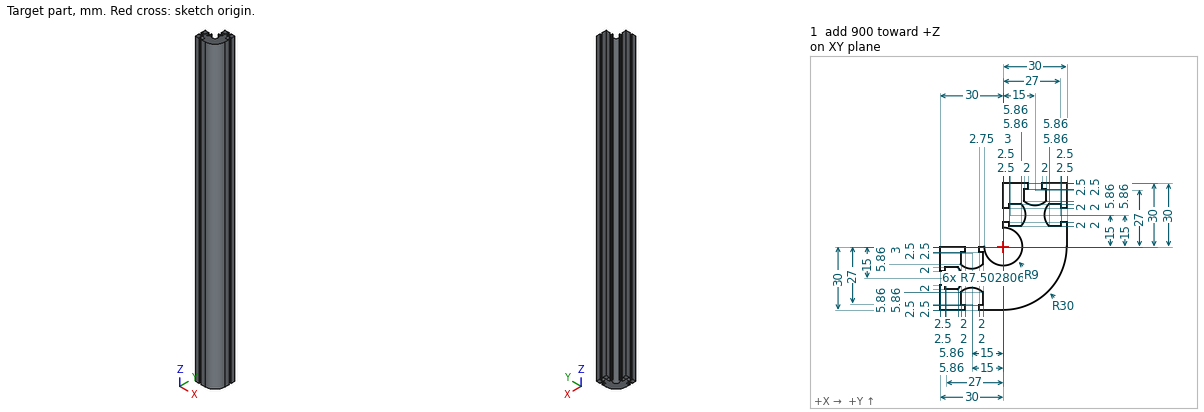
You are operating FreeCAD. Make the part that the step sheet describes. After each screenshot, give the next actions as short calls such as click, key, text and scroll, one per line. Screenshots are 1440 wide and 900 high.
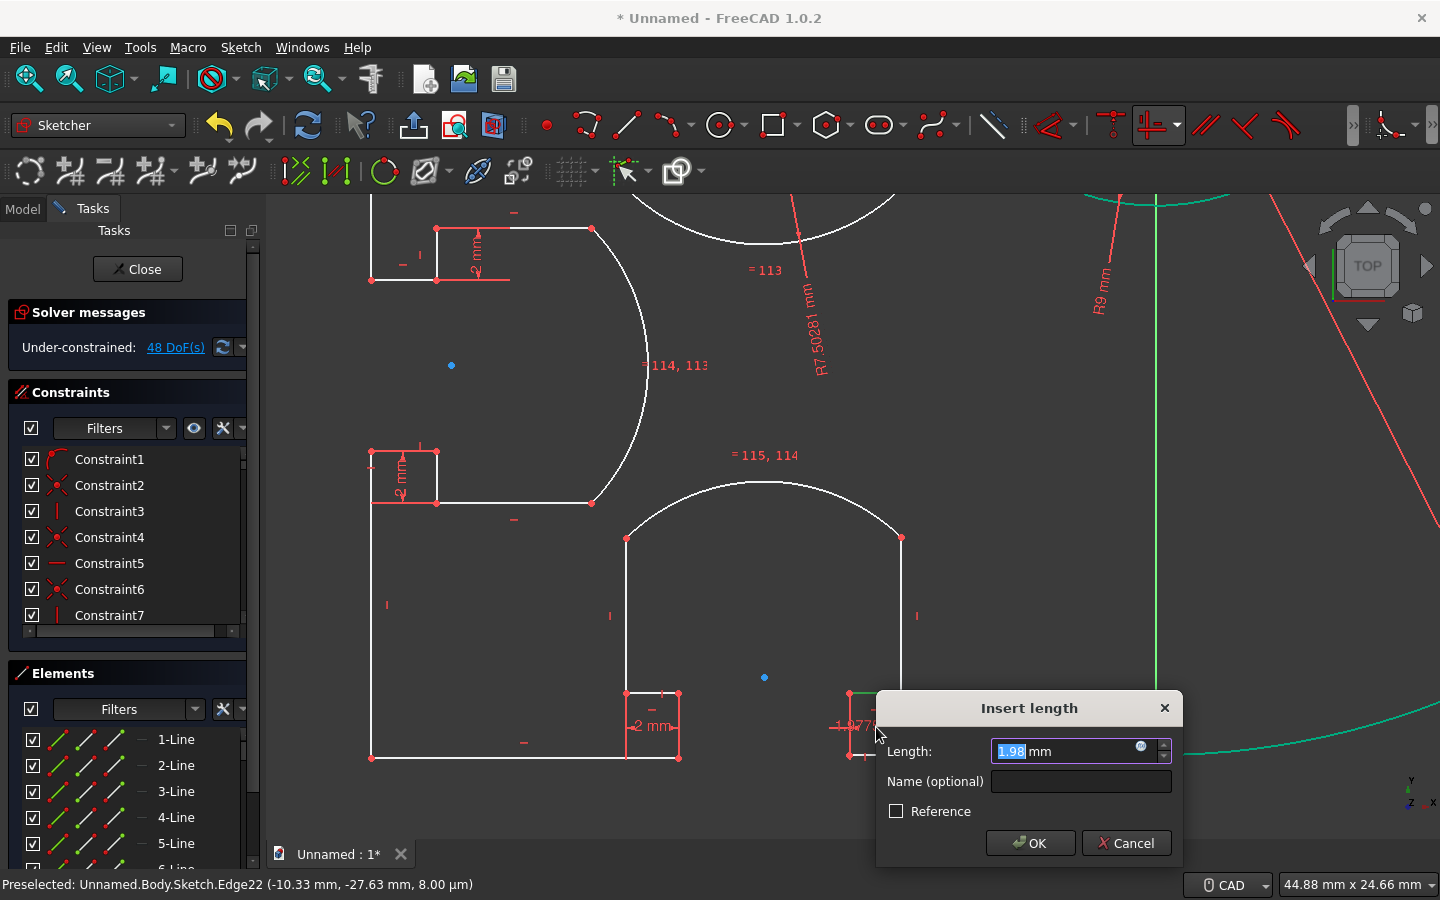
text(2)
key(Return)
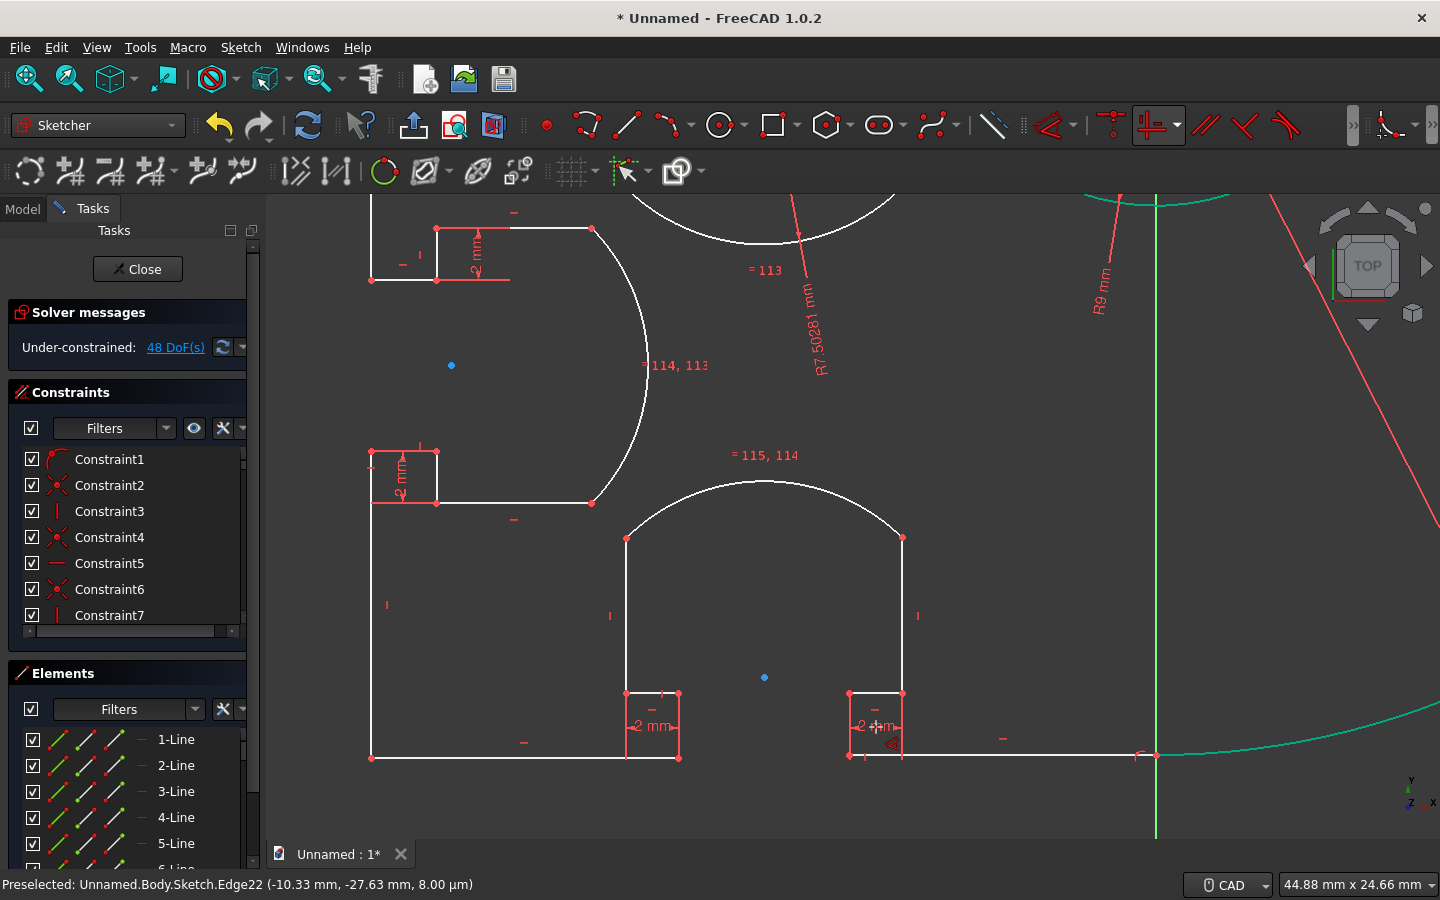
scroll(663, 695, down, 7)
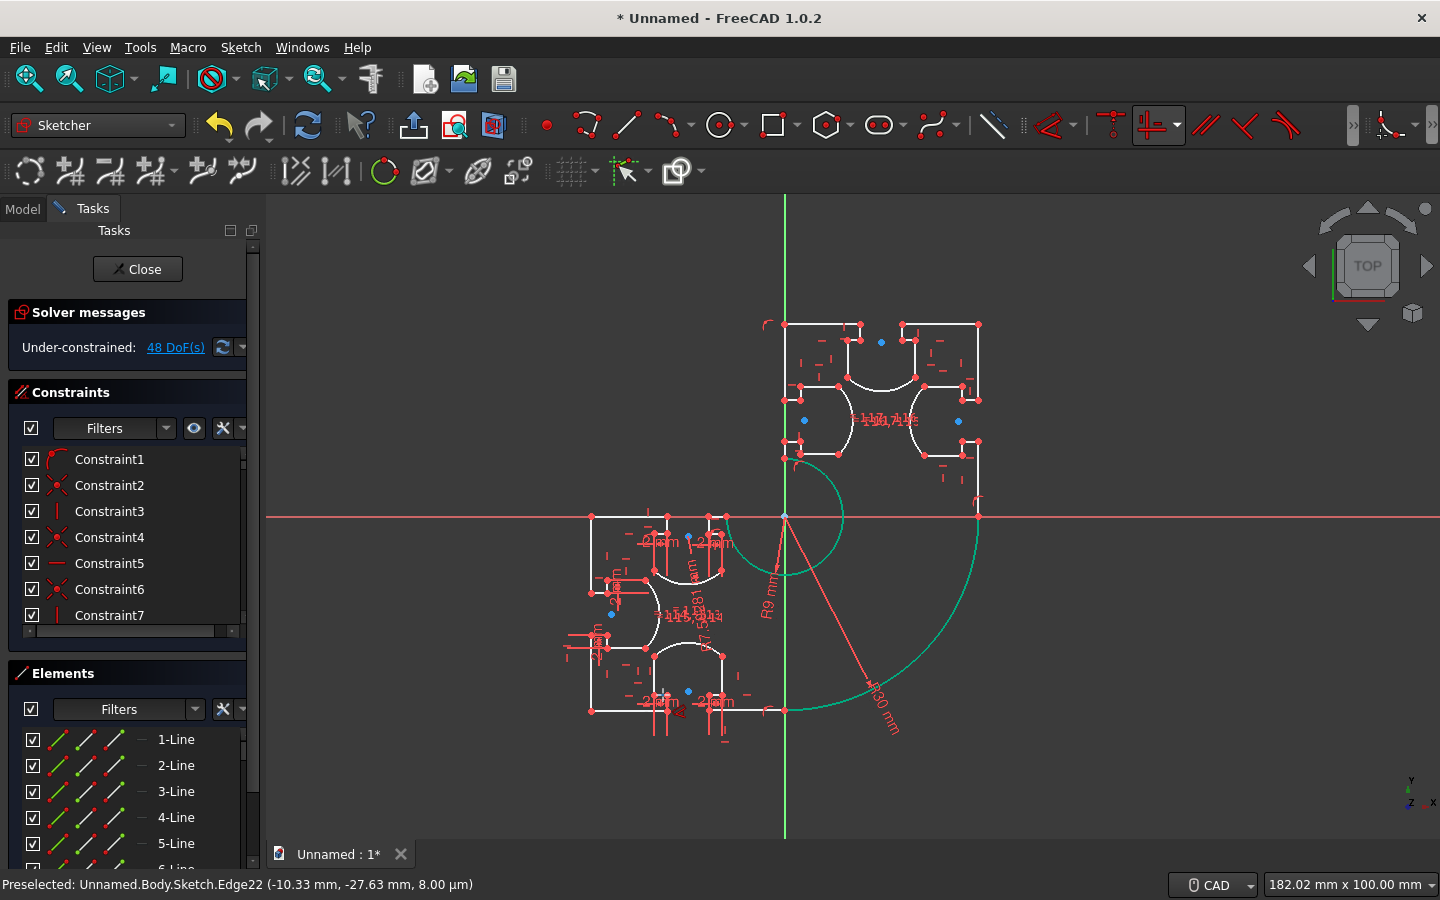
scroll(962, 446, up, 6)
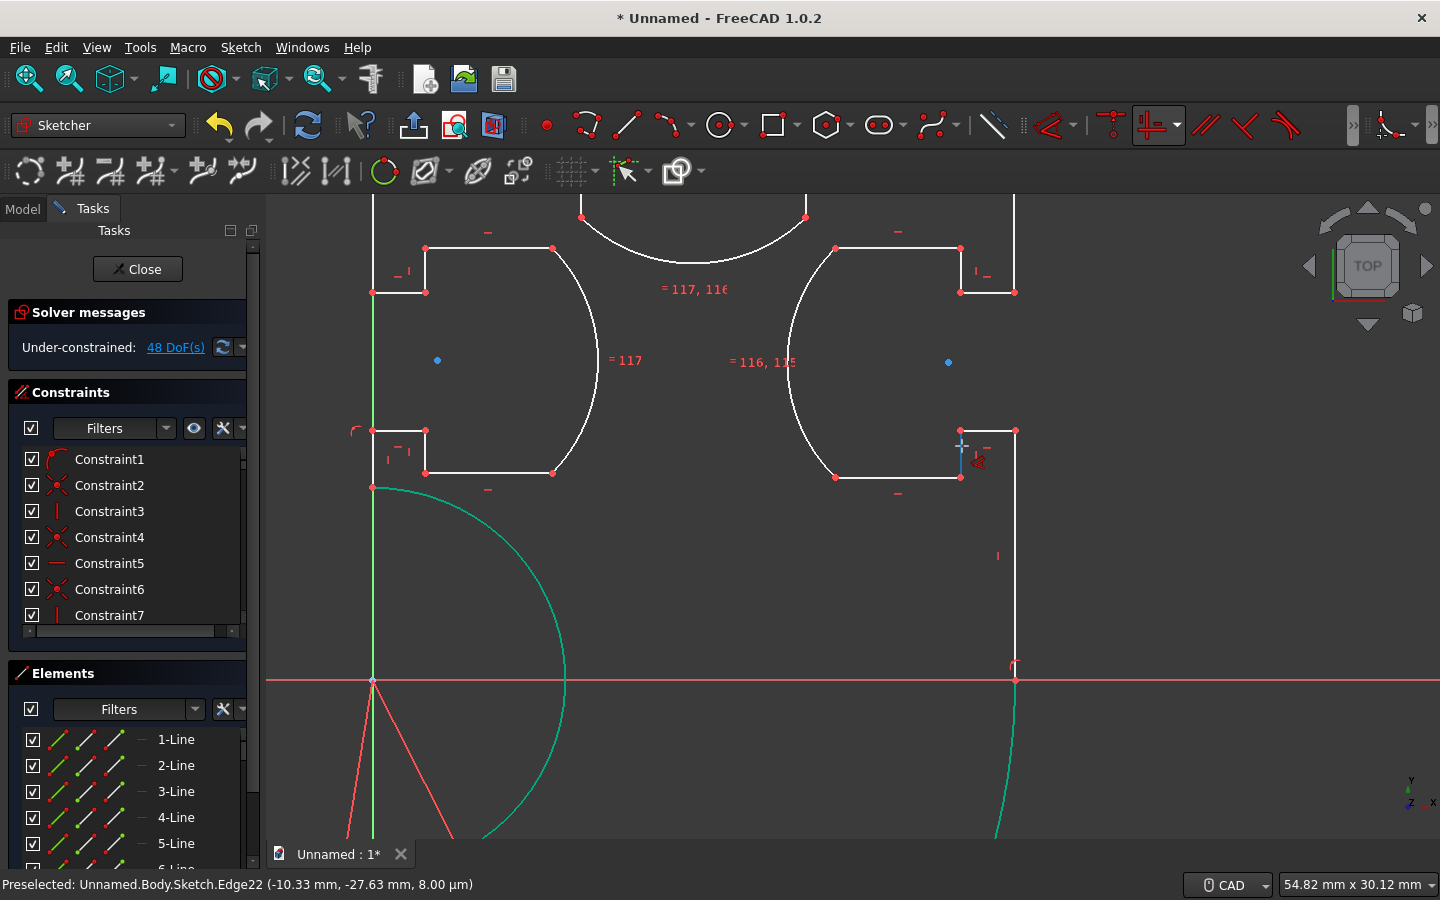
click(961, 445)
click(995, 454)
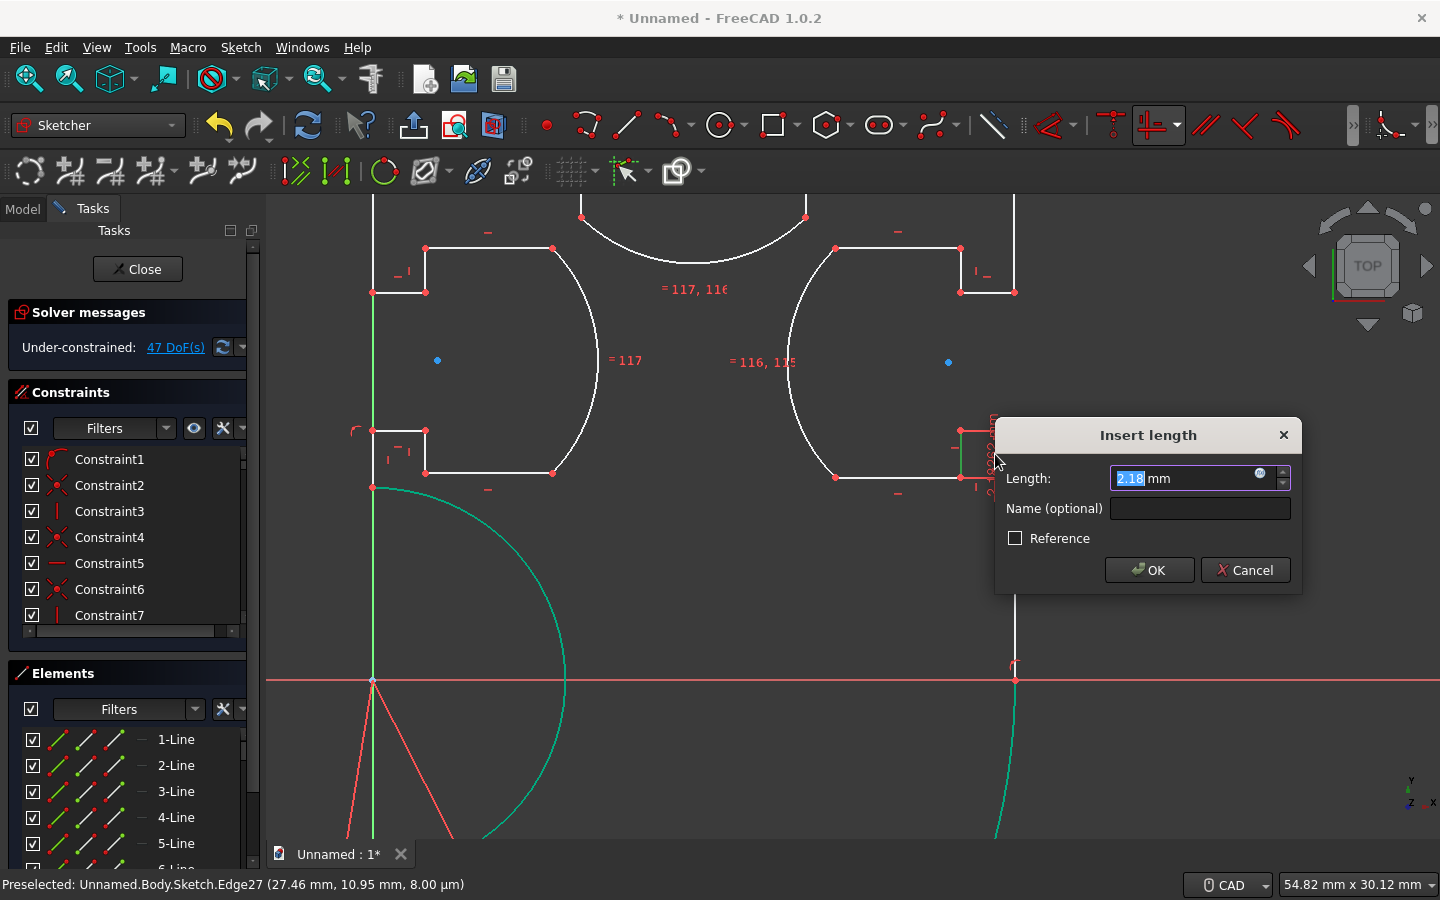
text(2)
key(Return)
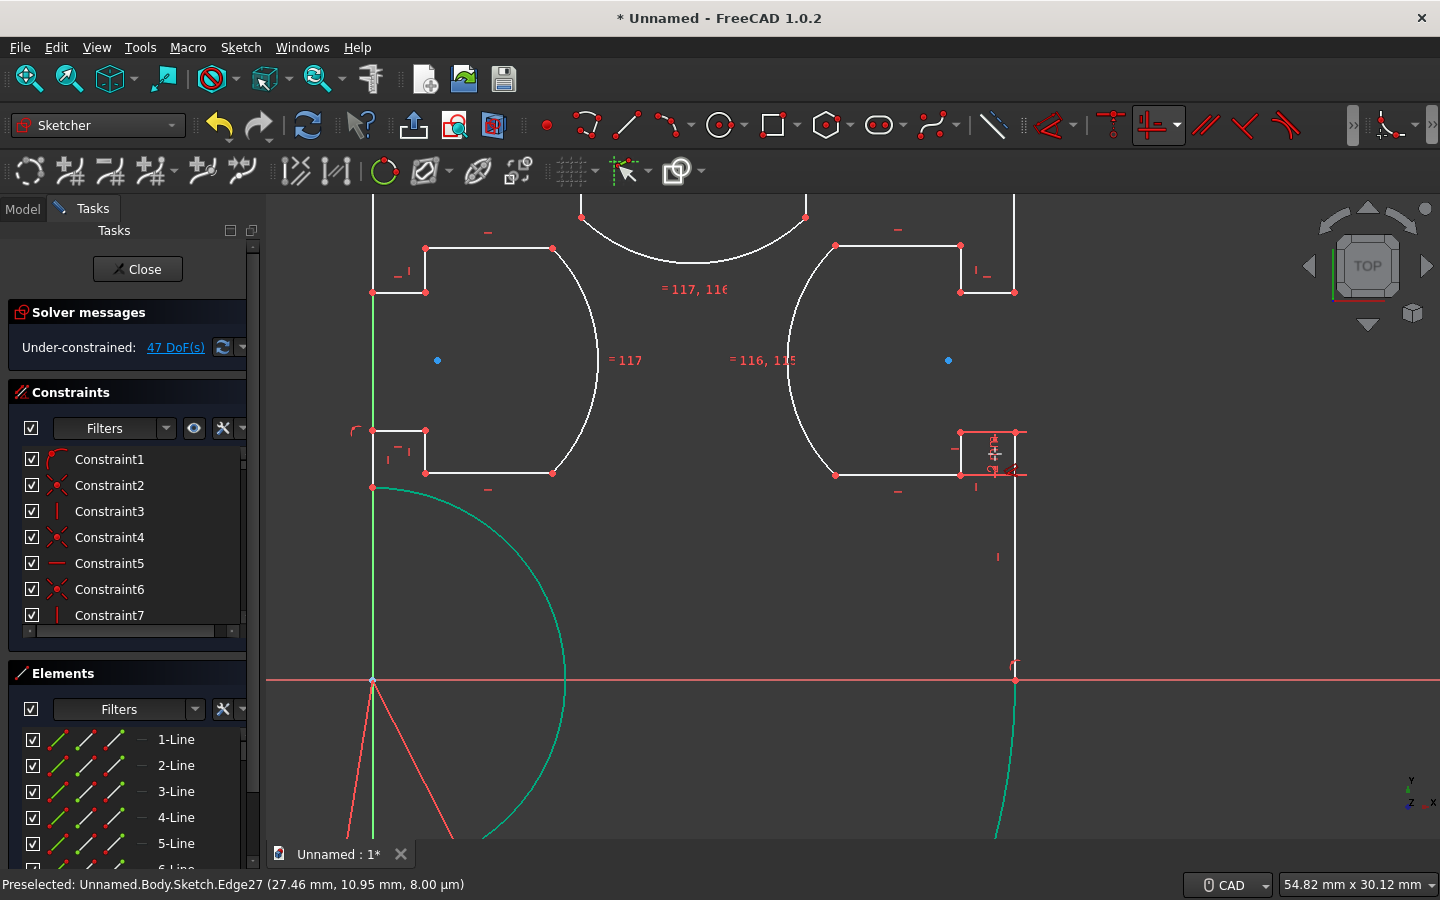
click(961, 260)
click(995, 269)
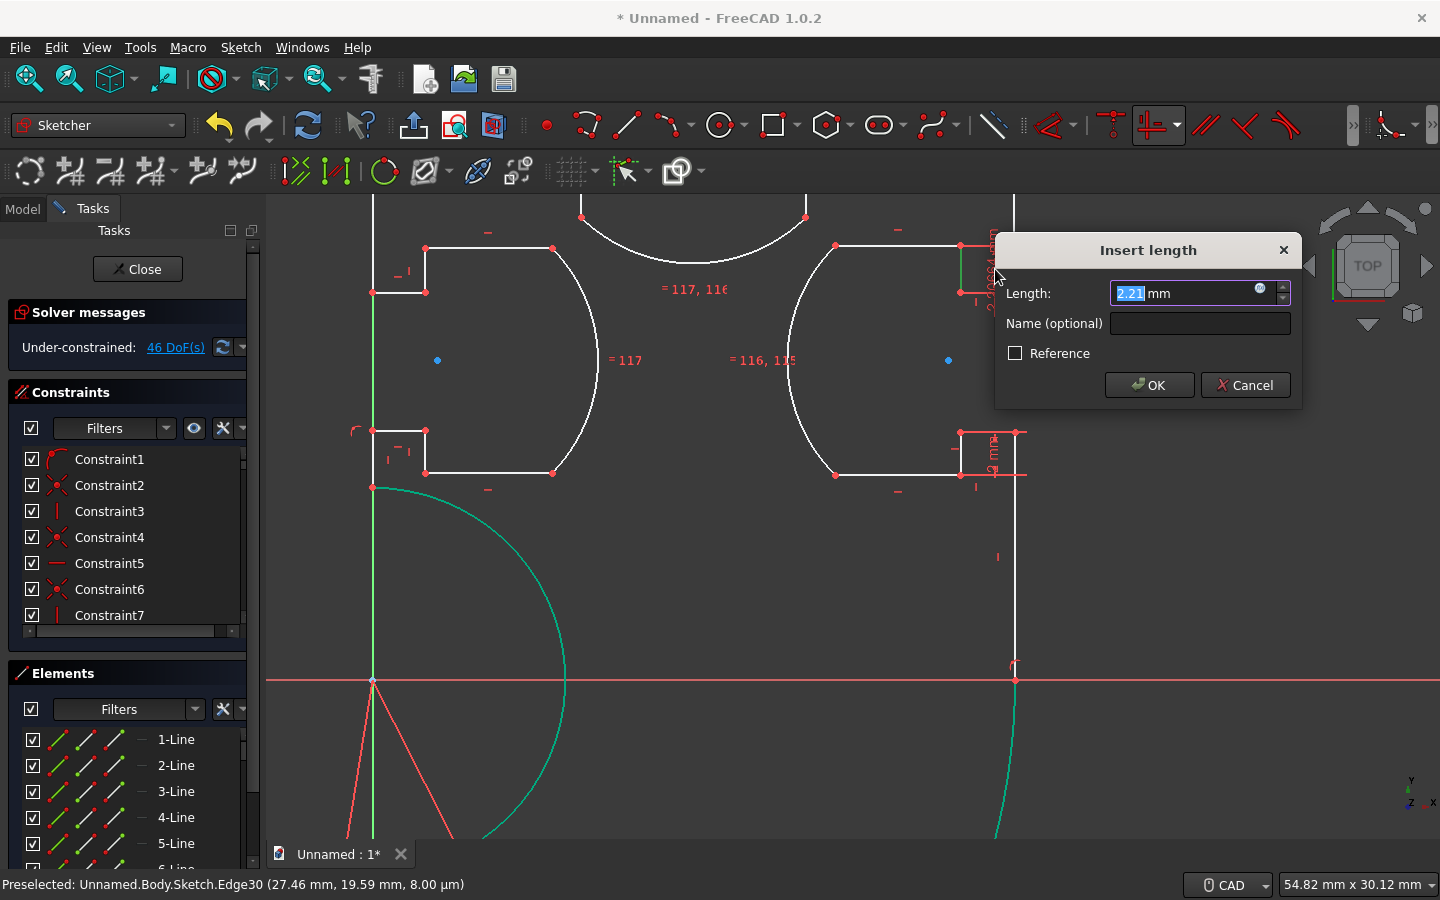
text(2)
key(Return)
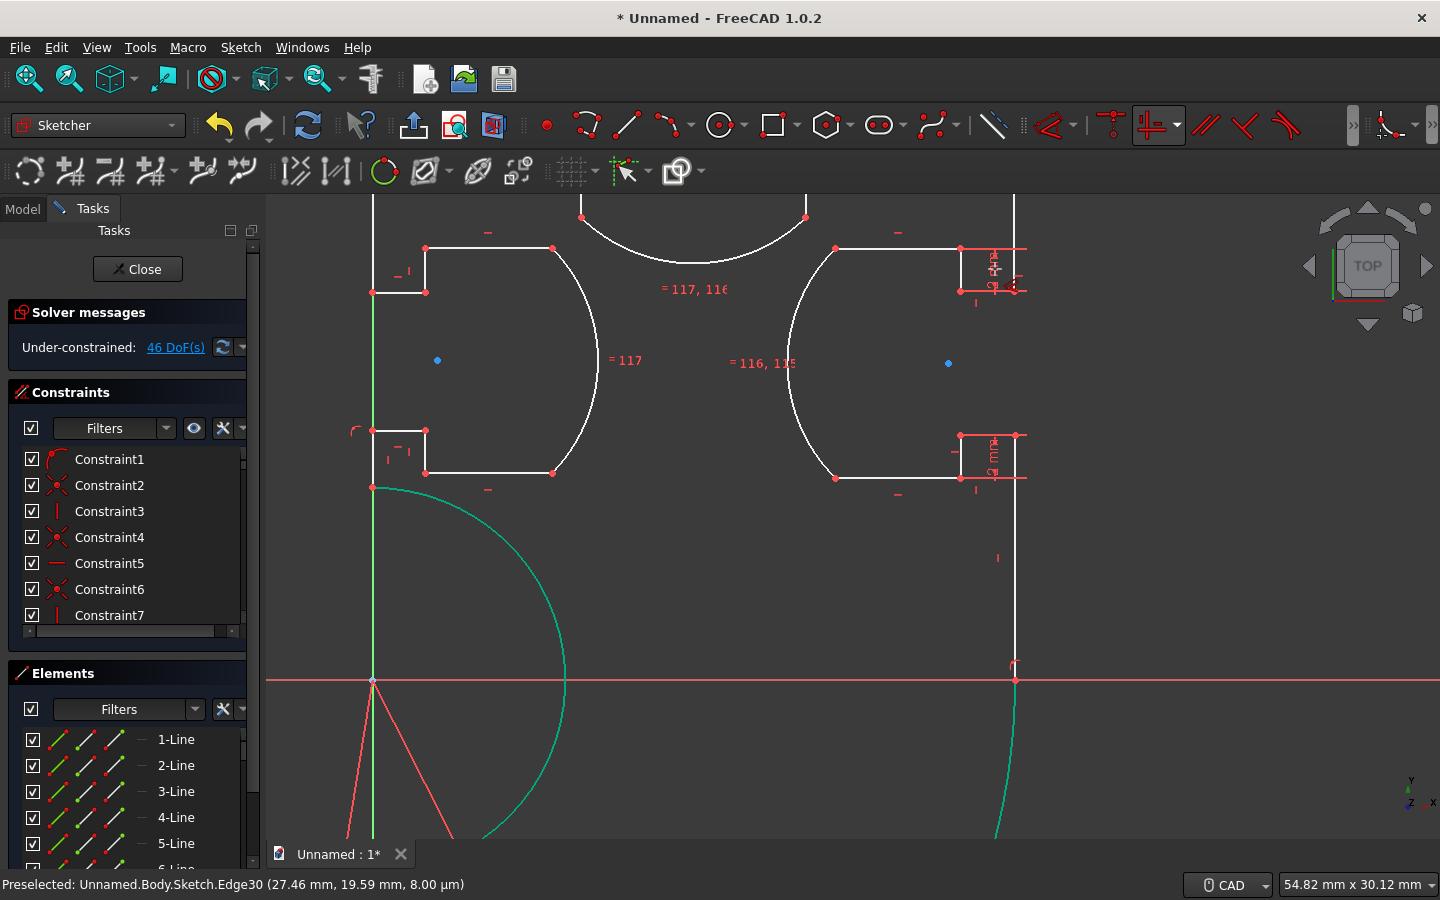
scroll(962, 446, down, 6)